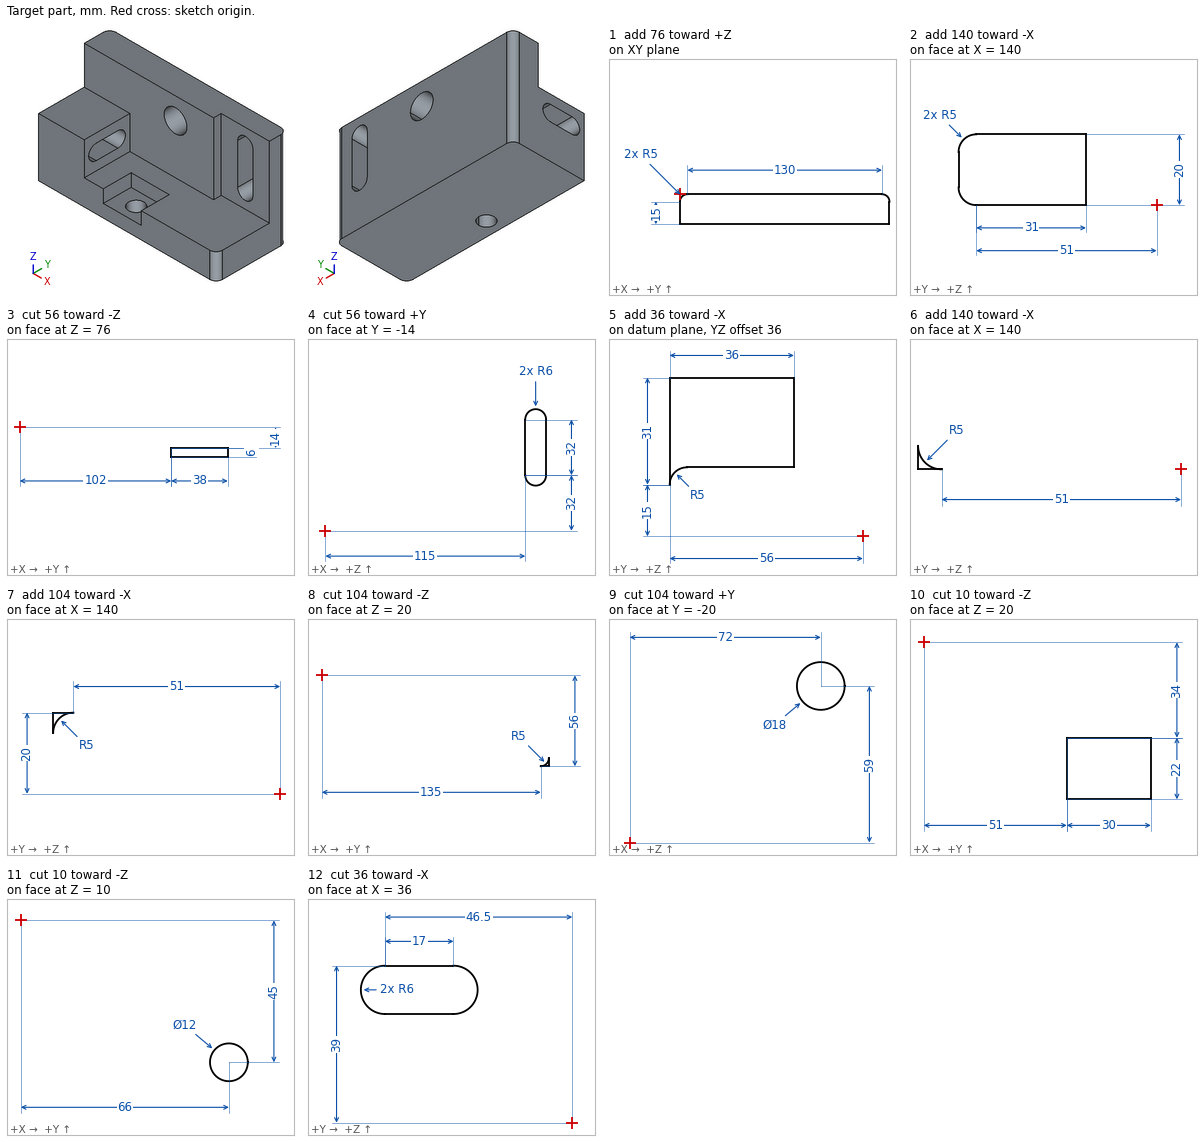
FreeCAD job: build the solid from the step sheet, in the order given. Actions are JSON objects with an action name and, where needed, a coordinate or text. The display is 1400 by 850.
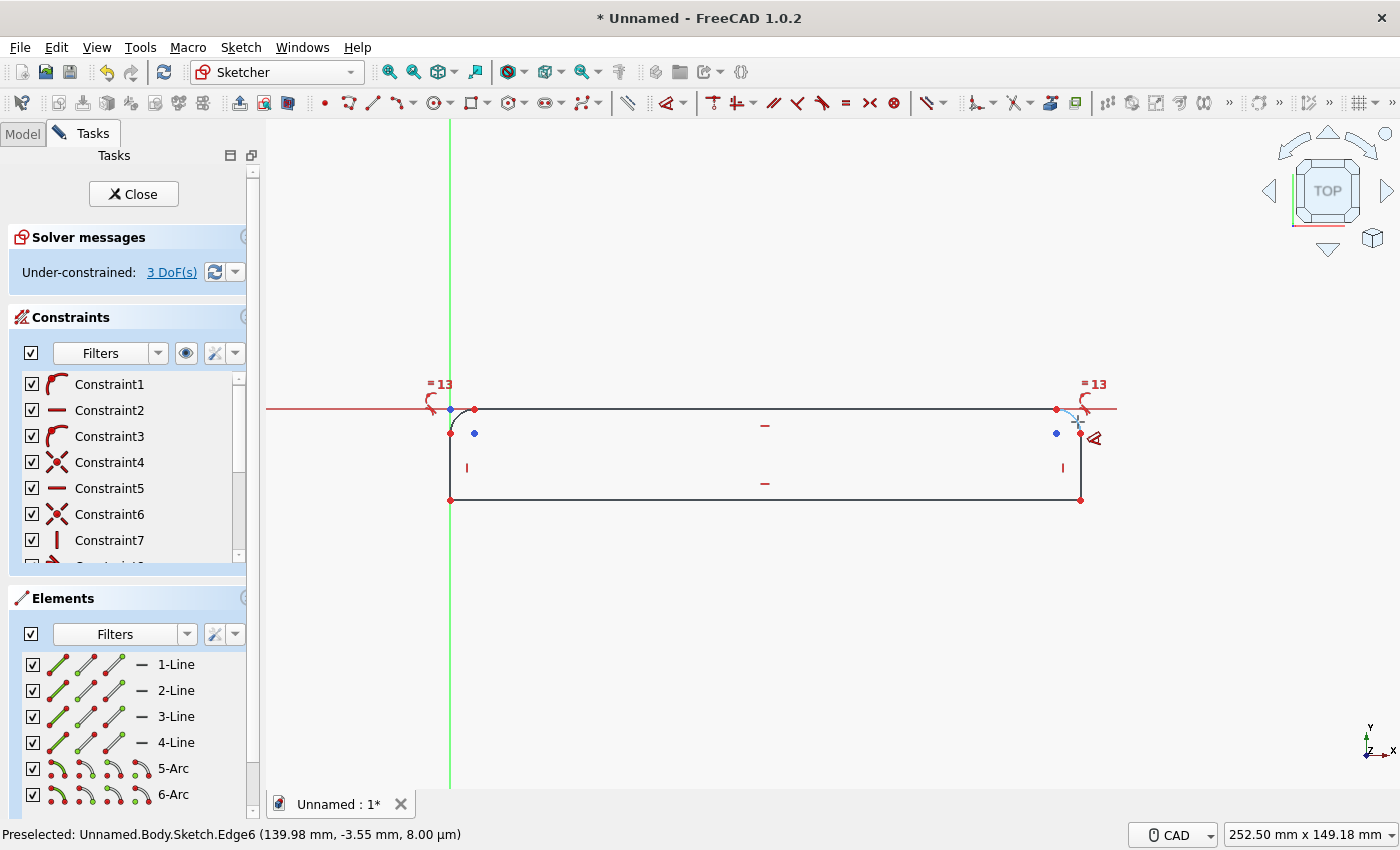
{"action": "scroll", "coordinate": [464, 412], "scroll_direction": "up", "scroll_amount": 3}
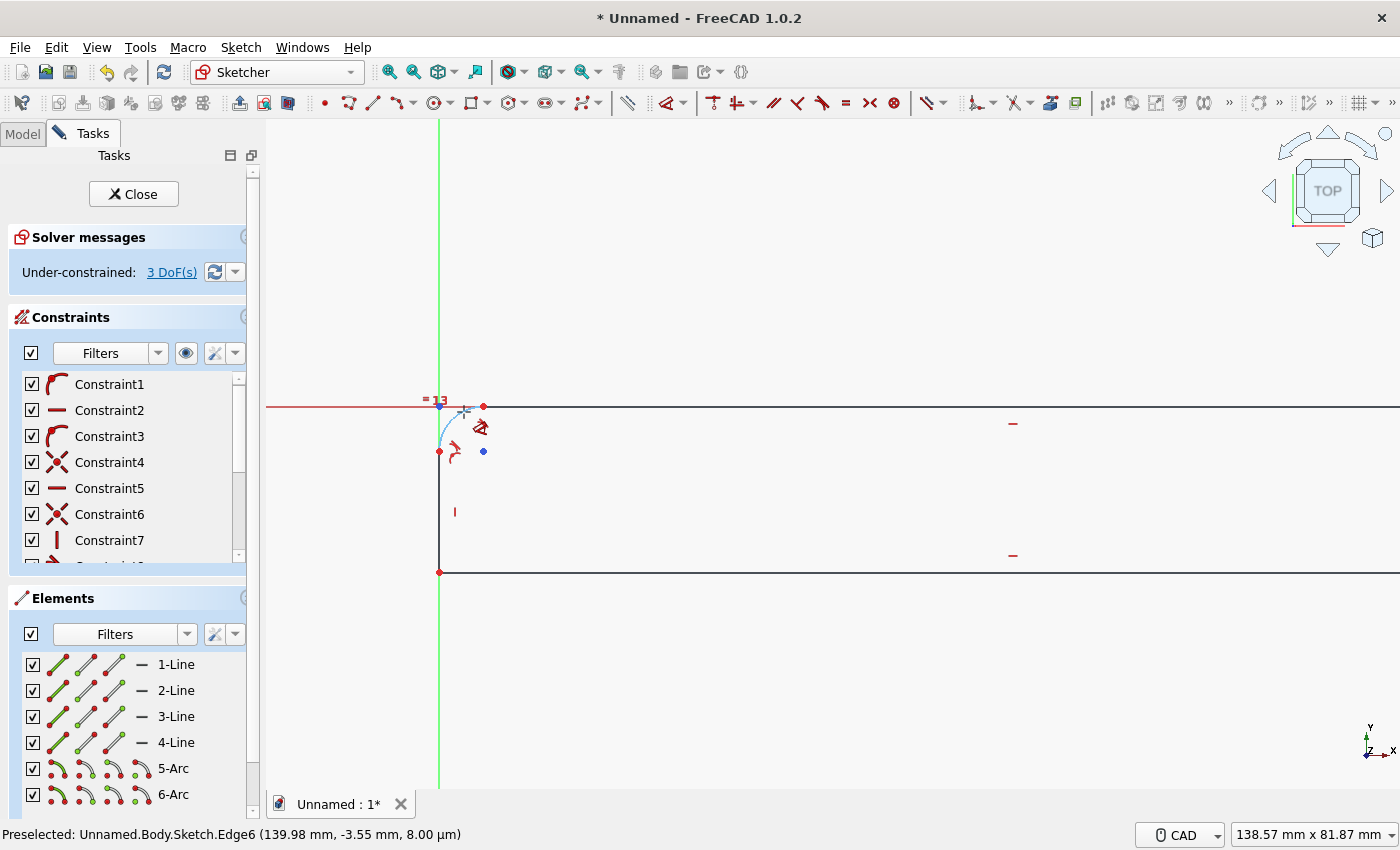
{"action": "left_click", "coordinate": [464, 411]}
{"action": "left_click", "coordinate": [487, 374]}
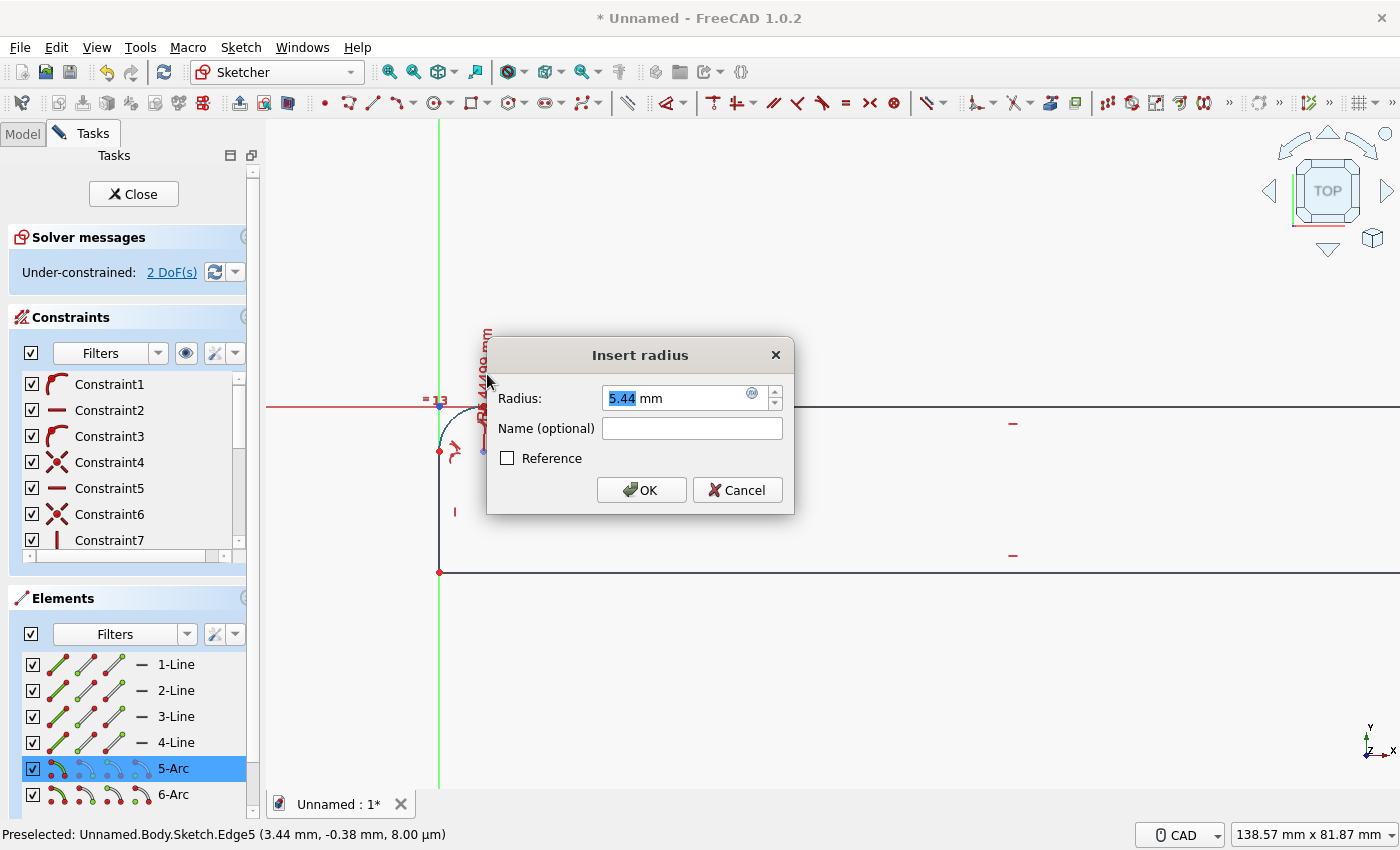
{"action": "type", "text": "5"}
{"action": "key", "text": "Return"}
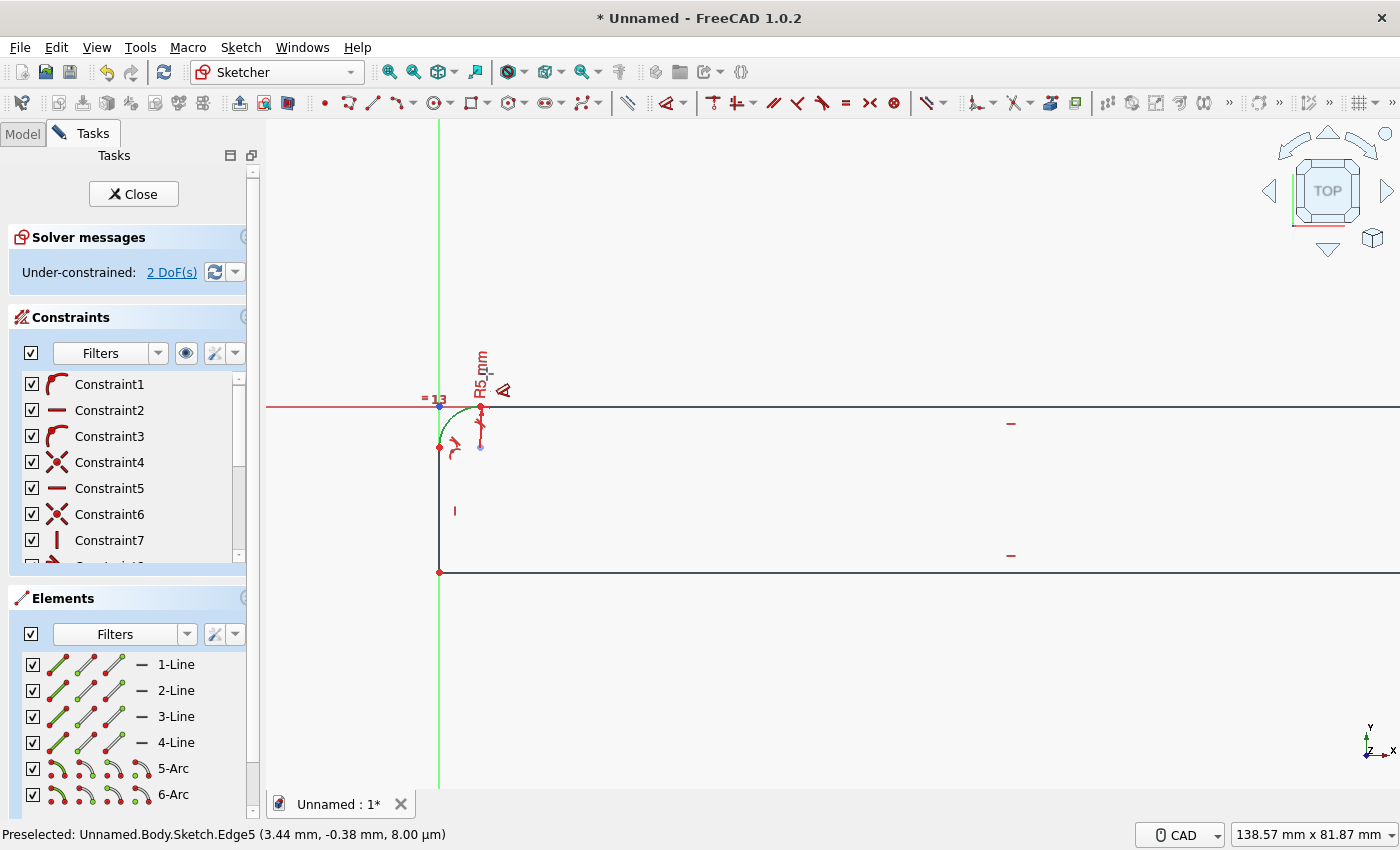
{"action": "left_click", "coordinate": [439, 485]}
{"action": "left_click", "coordinate": [405, 510]}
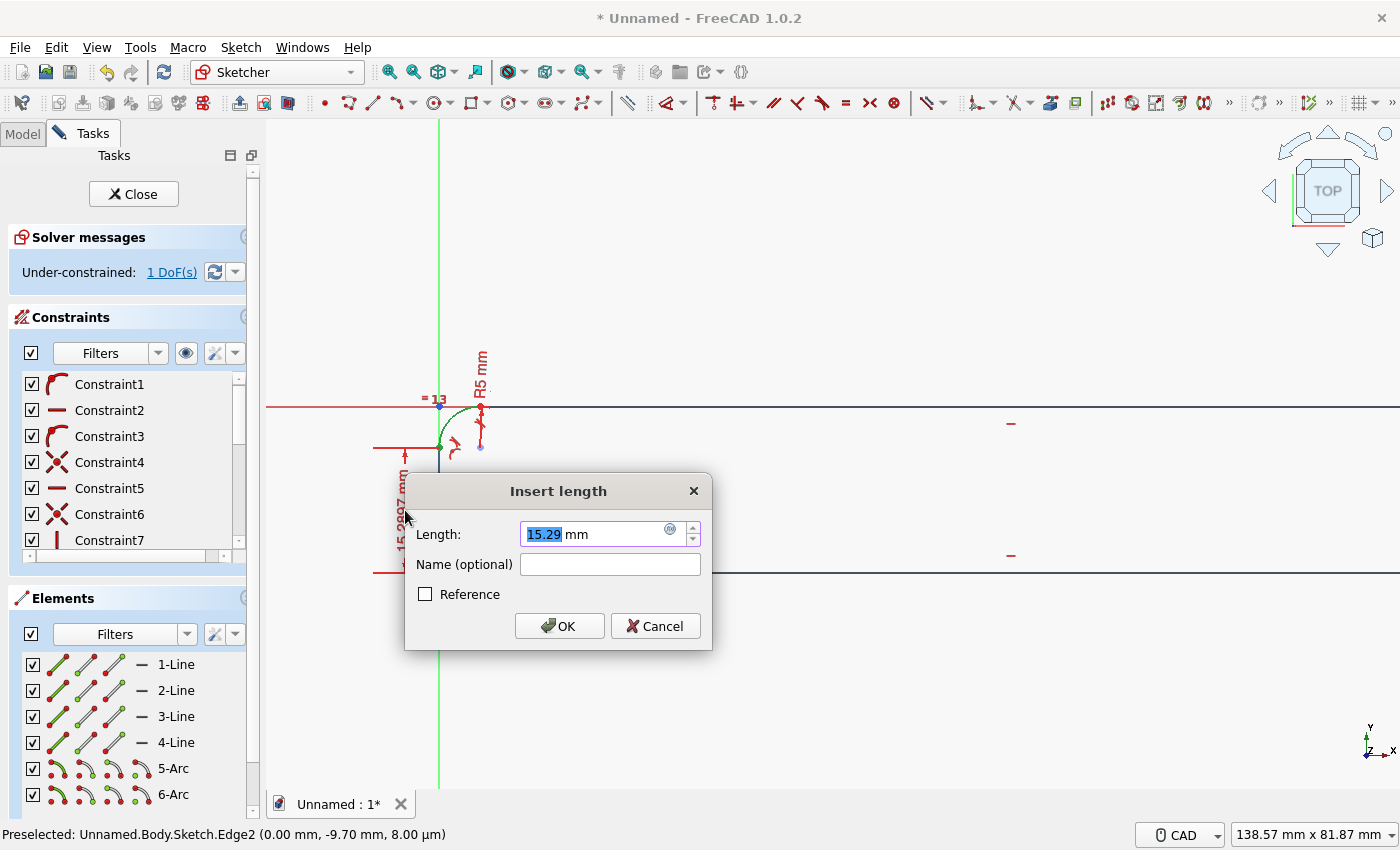
{"action": "type", "text": "15"}
{"action": "key", "text": "Return"}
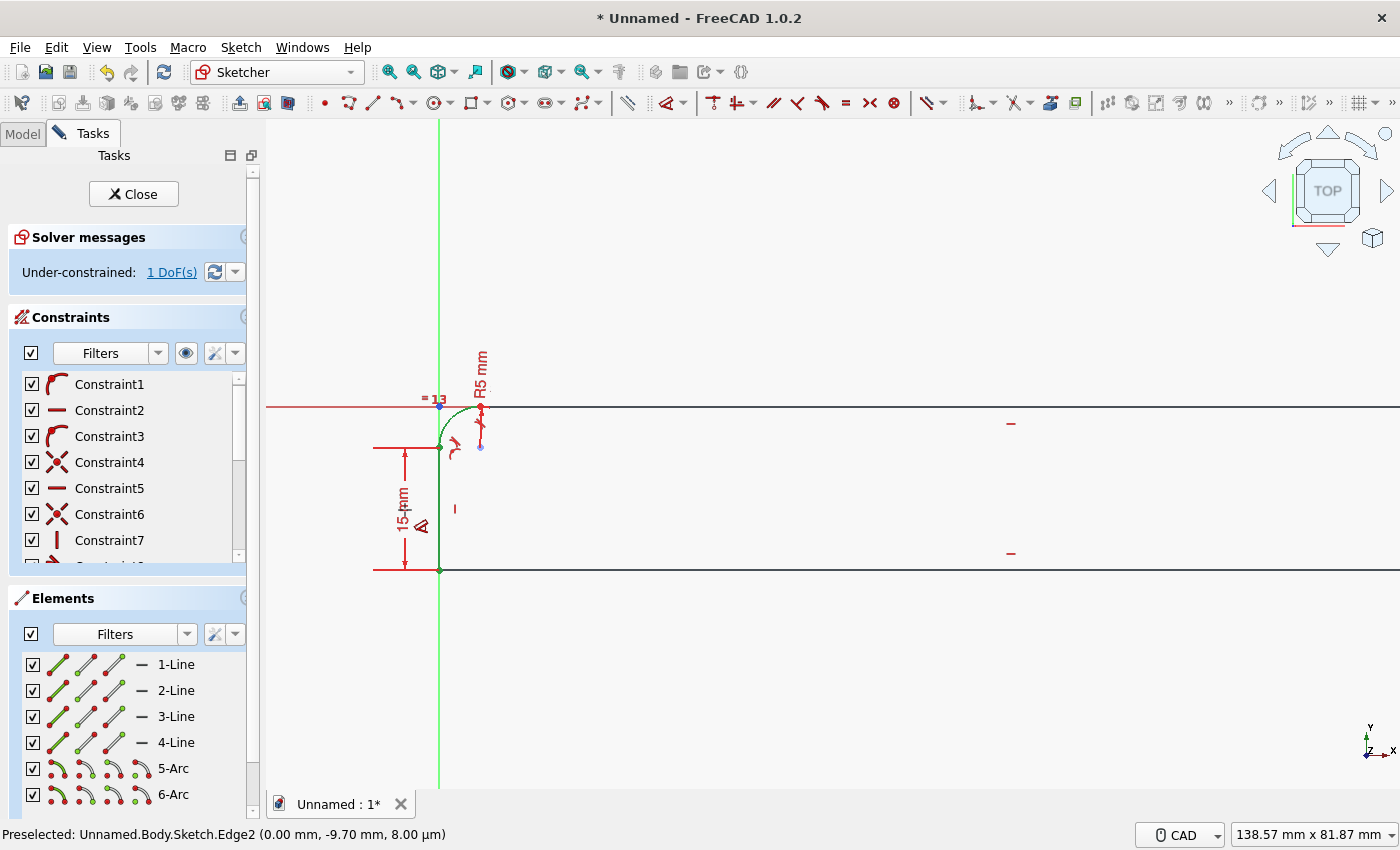
{"action": "left_click", "coordinate": [1224, 407]}
{"action": "left_click", "coordinate": [858, 373]}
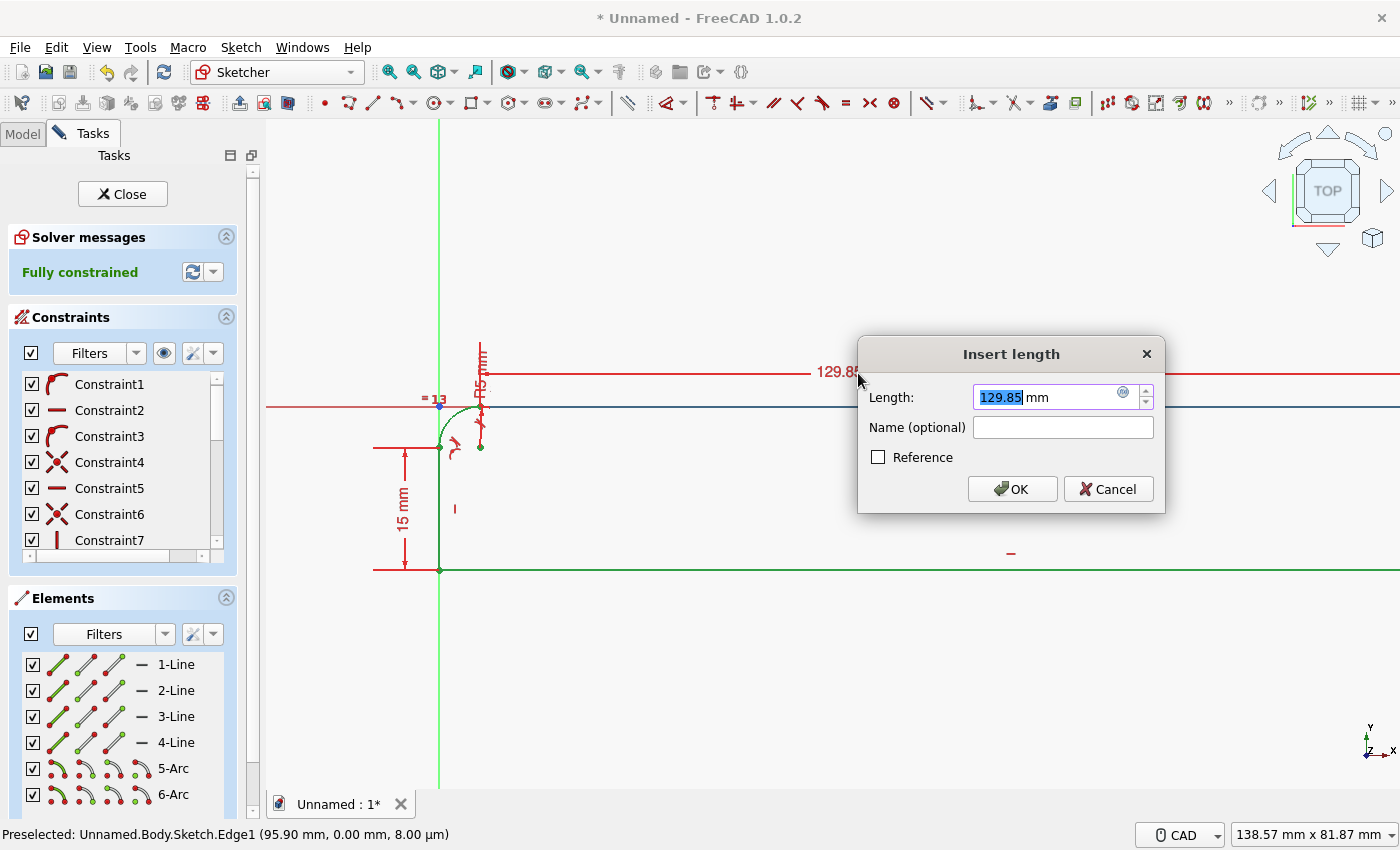
{"action": "type", "text": "130"}
{"action": "key", "text": "Return"}
{"action": "key", "text": "Escape"}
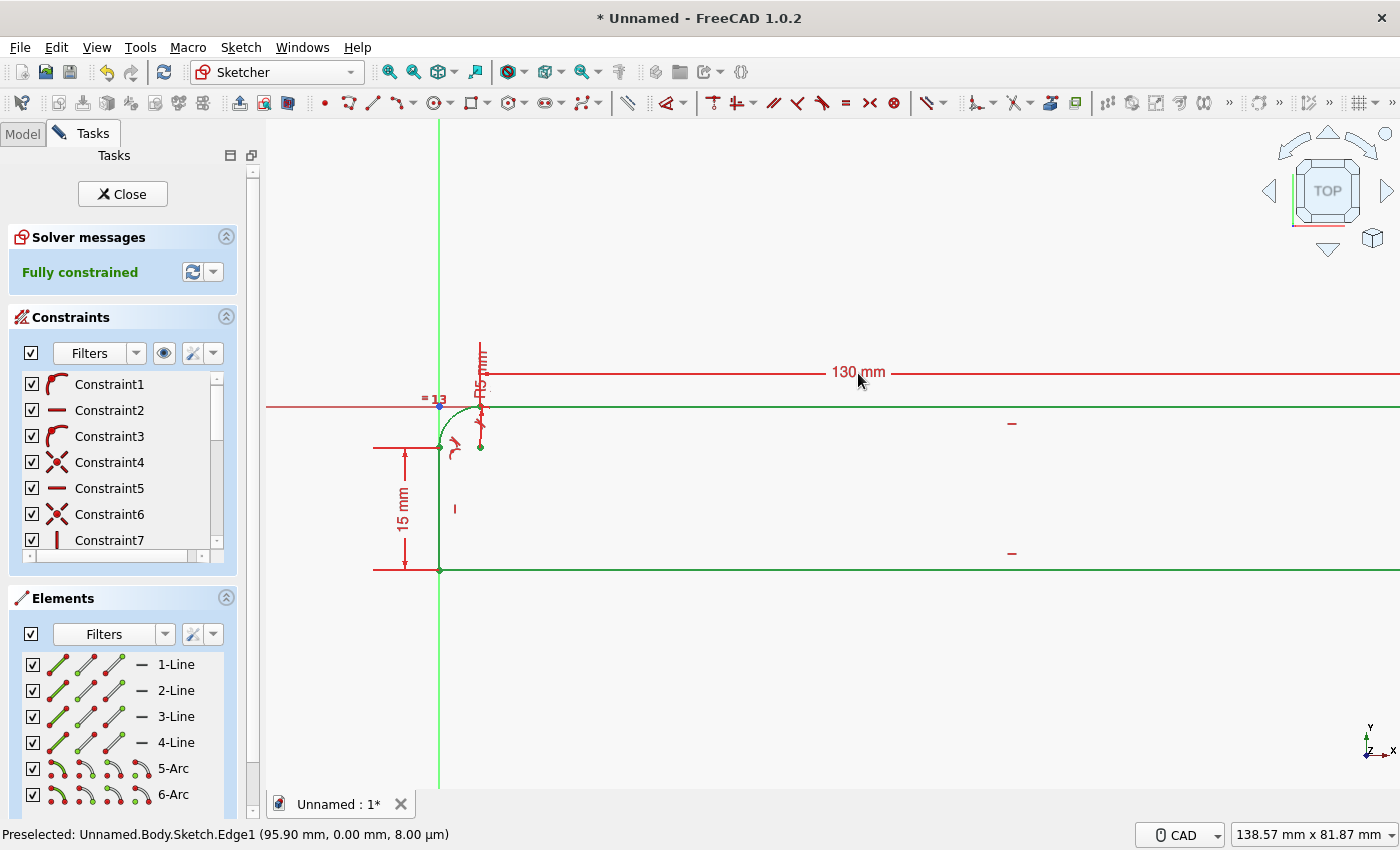
{"action": "left_click", "coordinate": [123, 194]}